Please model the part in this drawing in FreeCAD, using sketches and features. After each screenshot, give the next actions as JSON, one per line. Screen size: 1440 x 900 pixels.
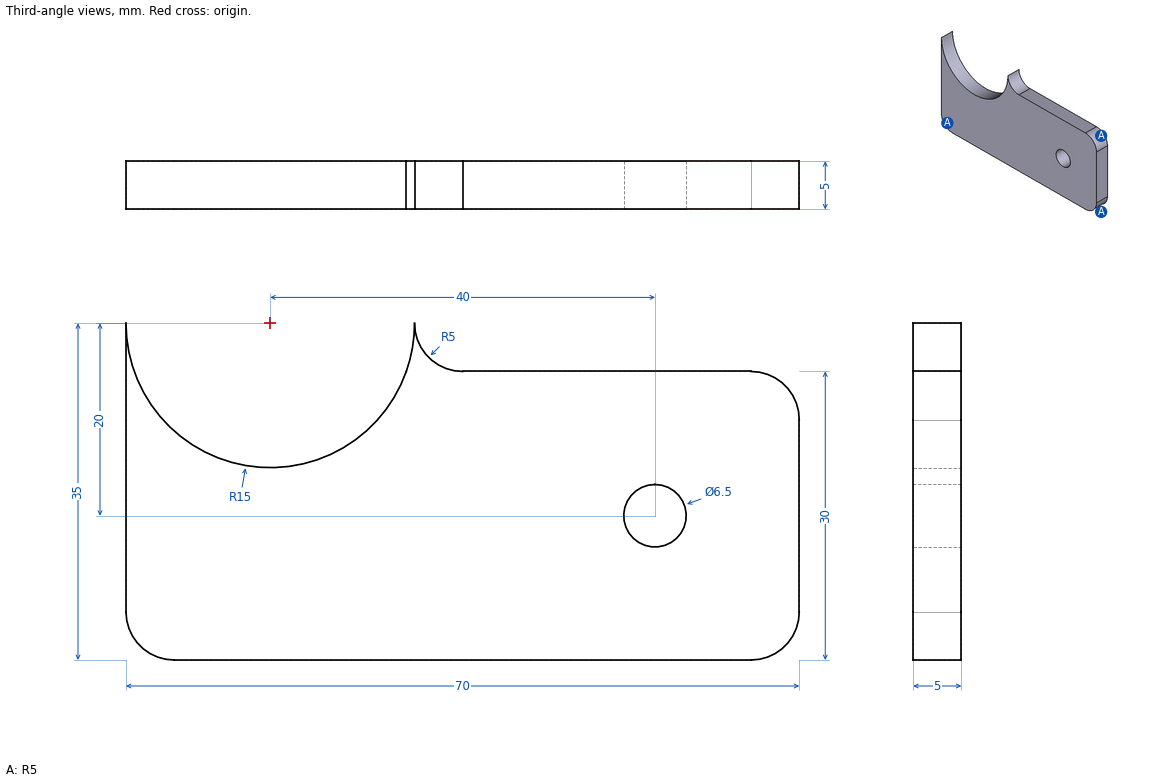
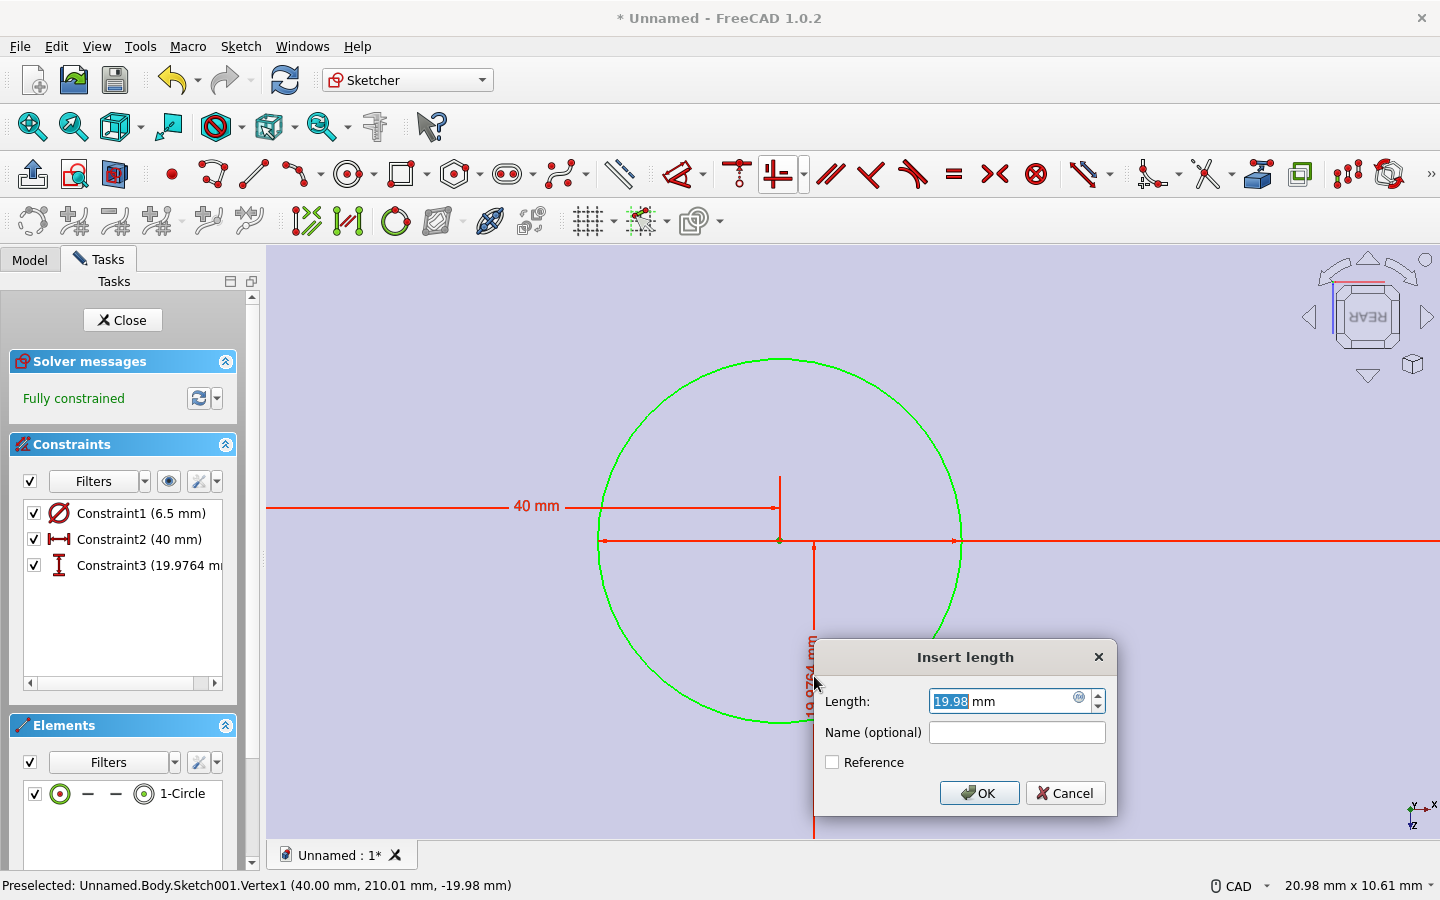
{"action": "type", "text": "20"}
{"action": "key", "text": "Return"}
{"action": "key", "text": "Escape"}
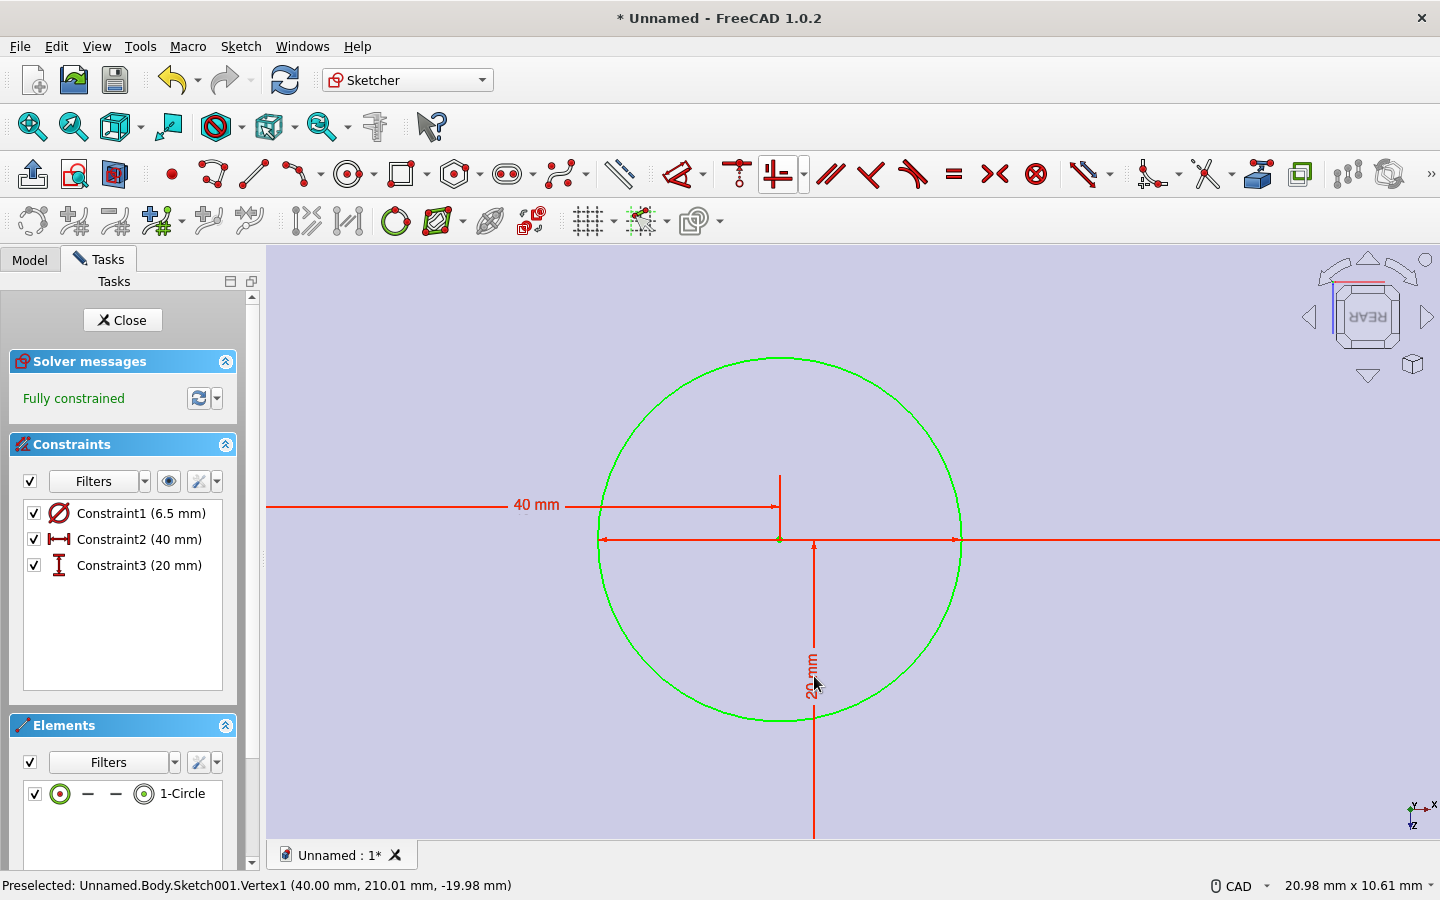
{"action": "left_click", "coordinate": [123, 320]}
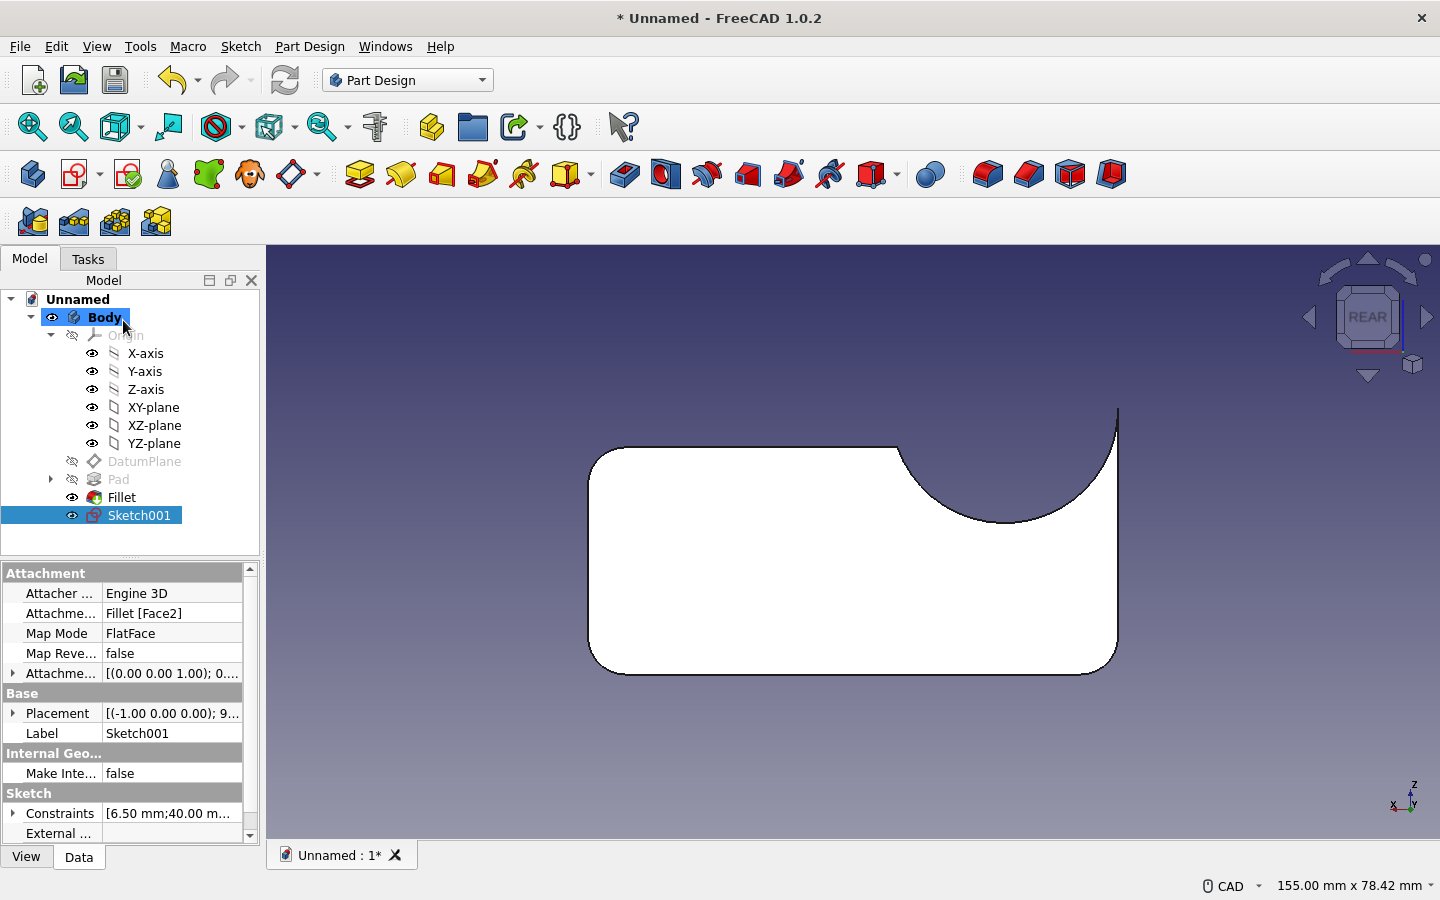
{"action": "left_click", "coordinate": [625, 174]}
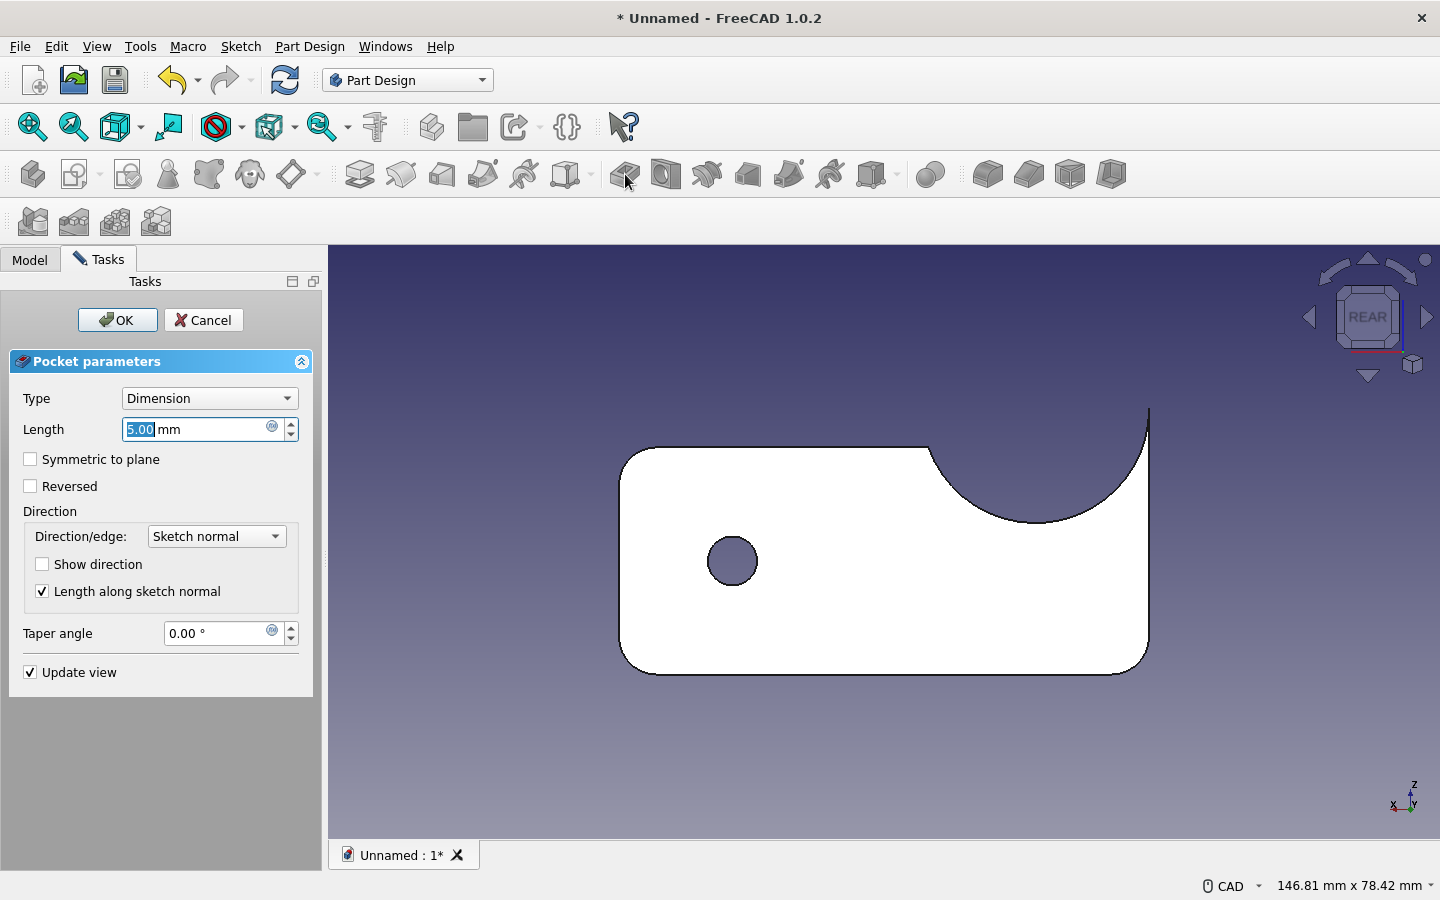
{"action": "type", "text": "5"}
{"action": "key", "text": "Tab"}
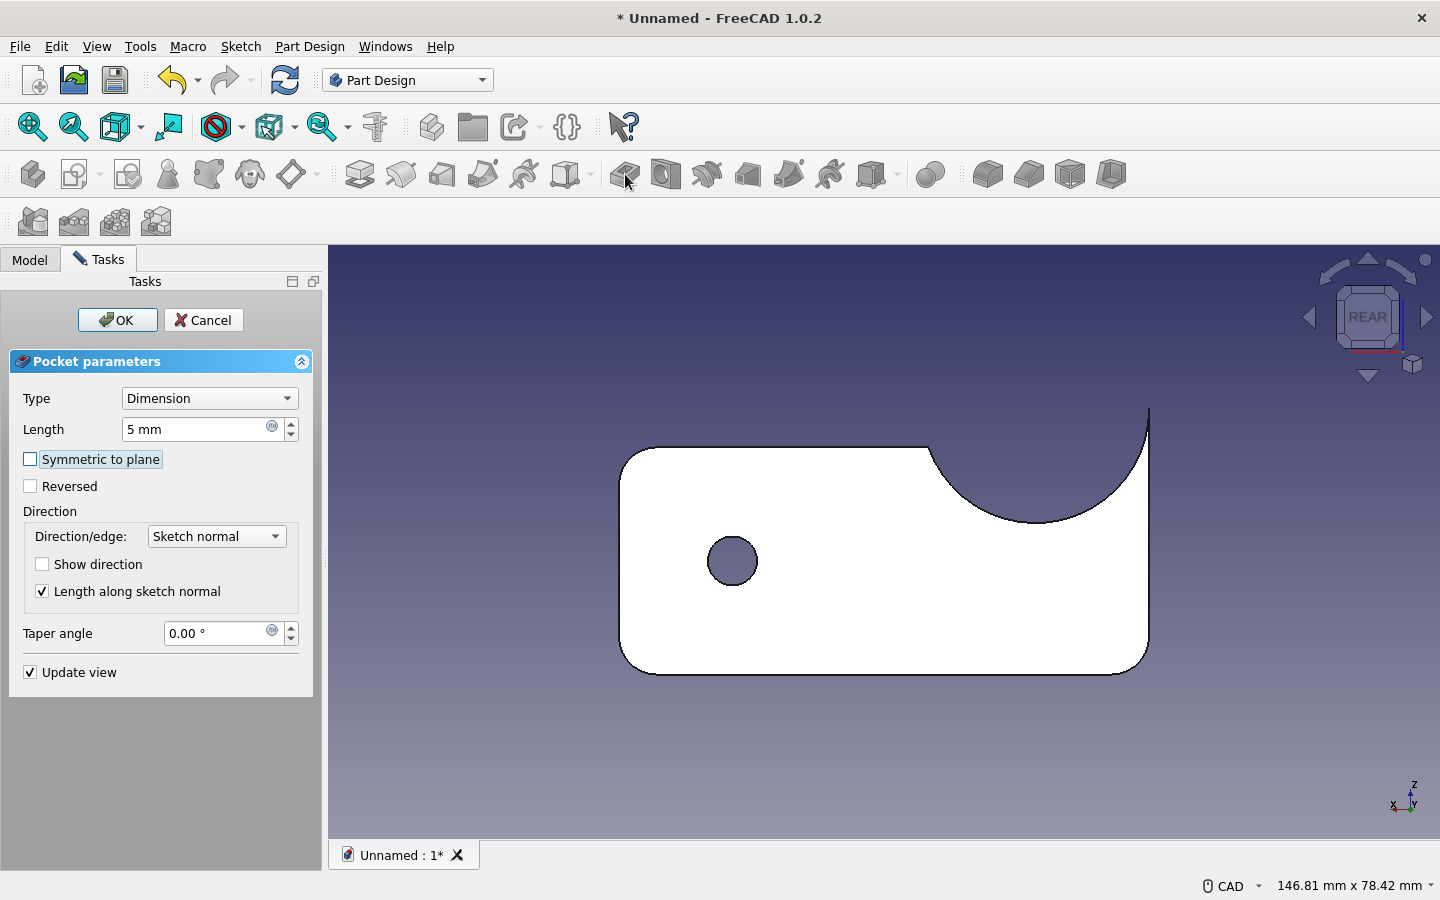
{"action": "left_click", "coordinate": [118, 320]}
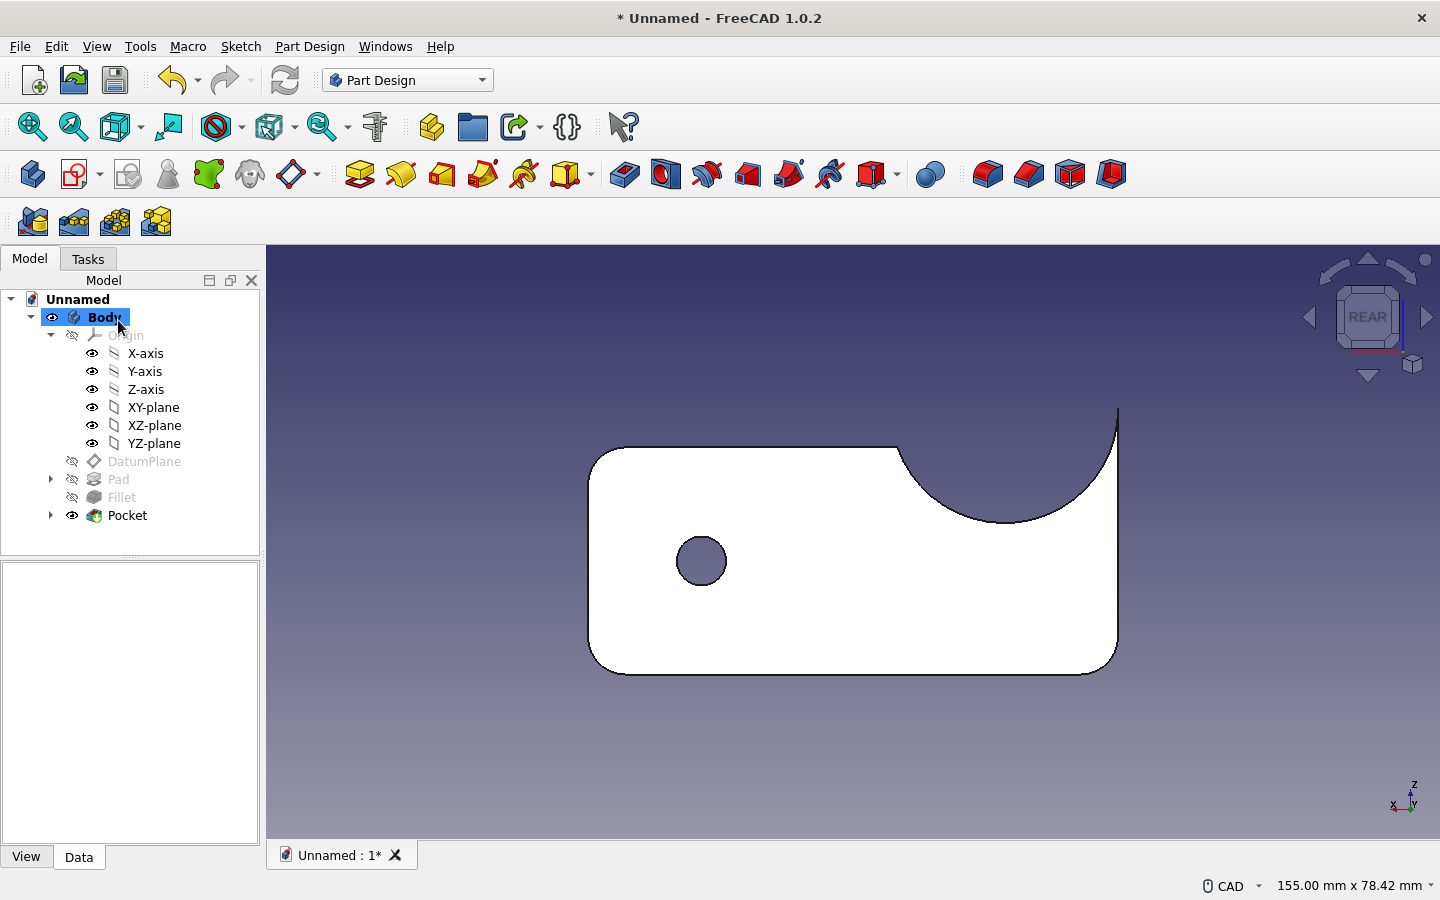
{"action": "left_click", "coordinate": [853, 579]}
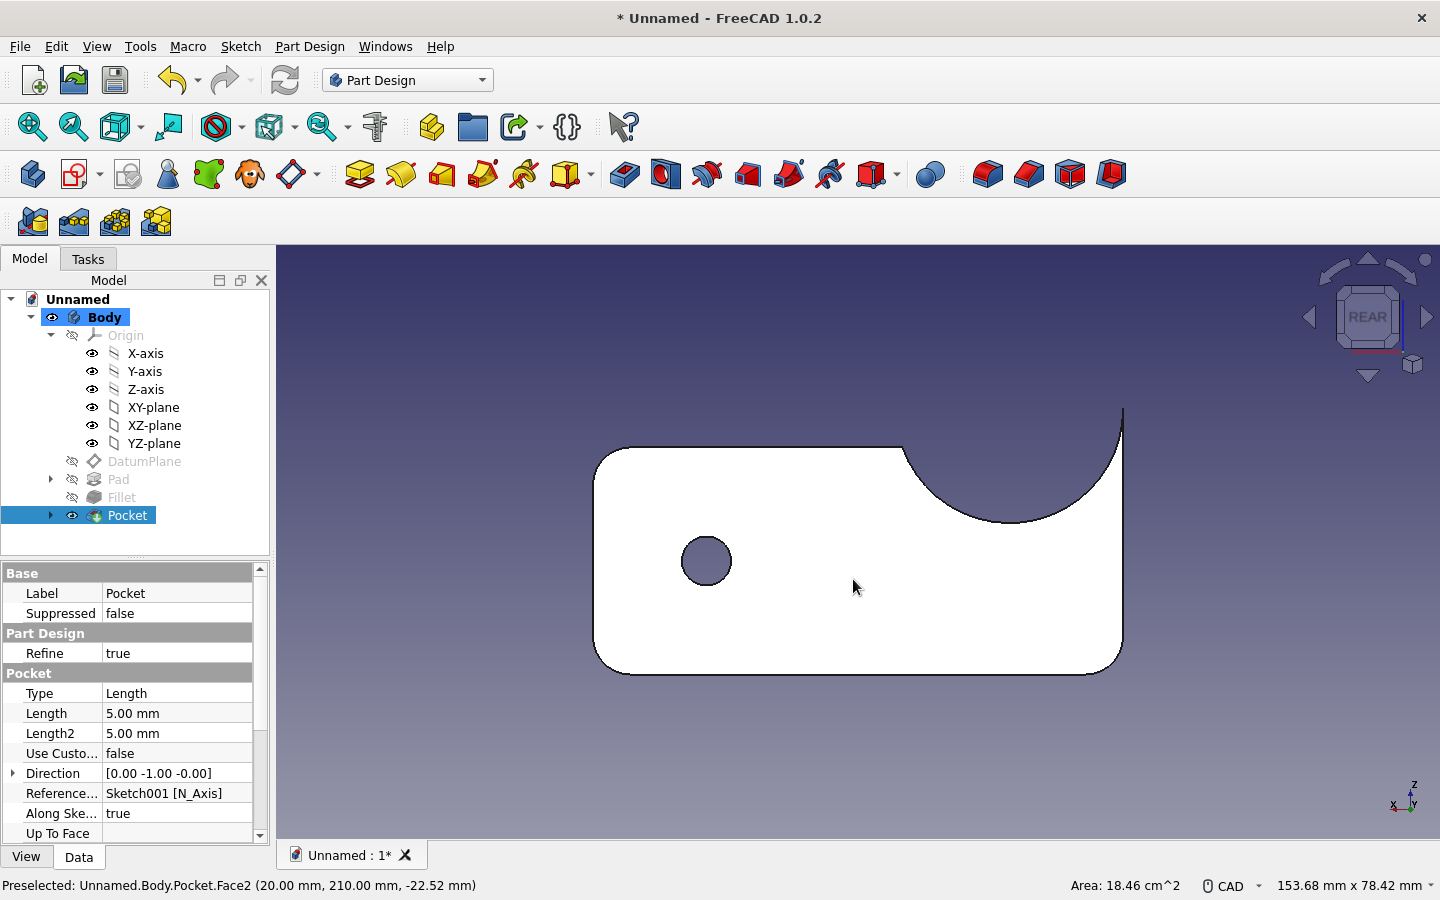
{"action": "left_click", "coordinate": [74, 174]}